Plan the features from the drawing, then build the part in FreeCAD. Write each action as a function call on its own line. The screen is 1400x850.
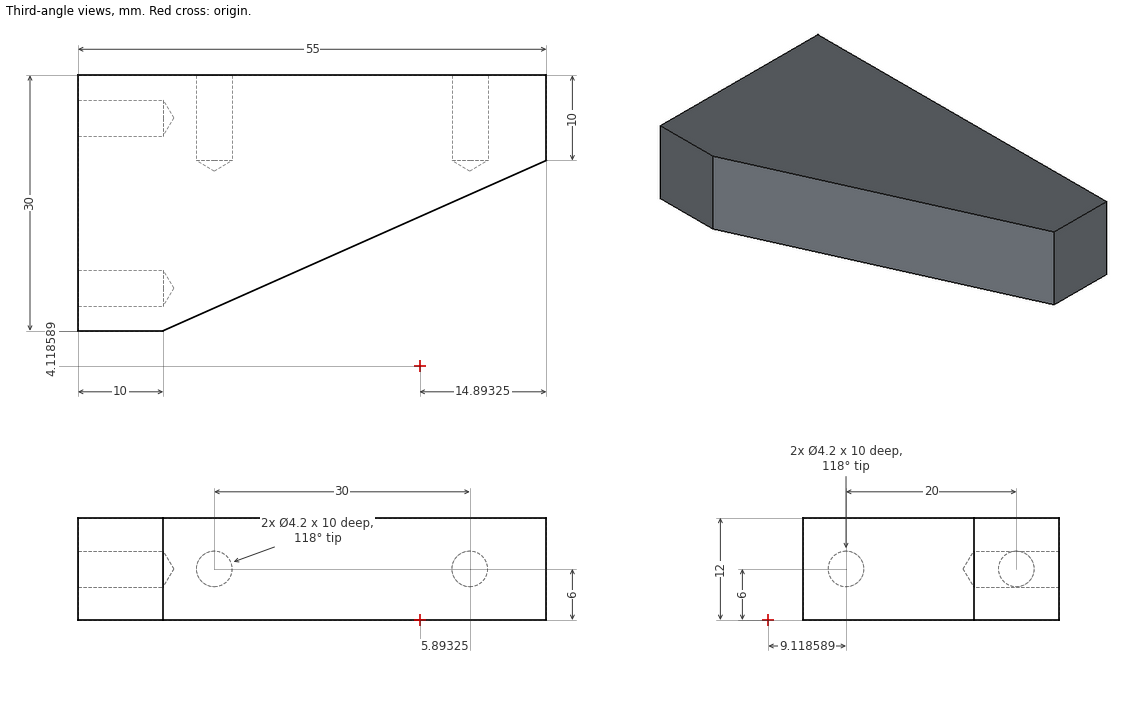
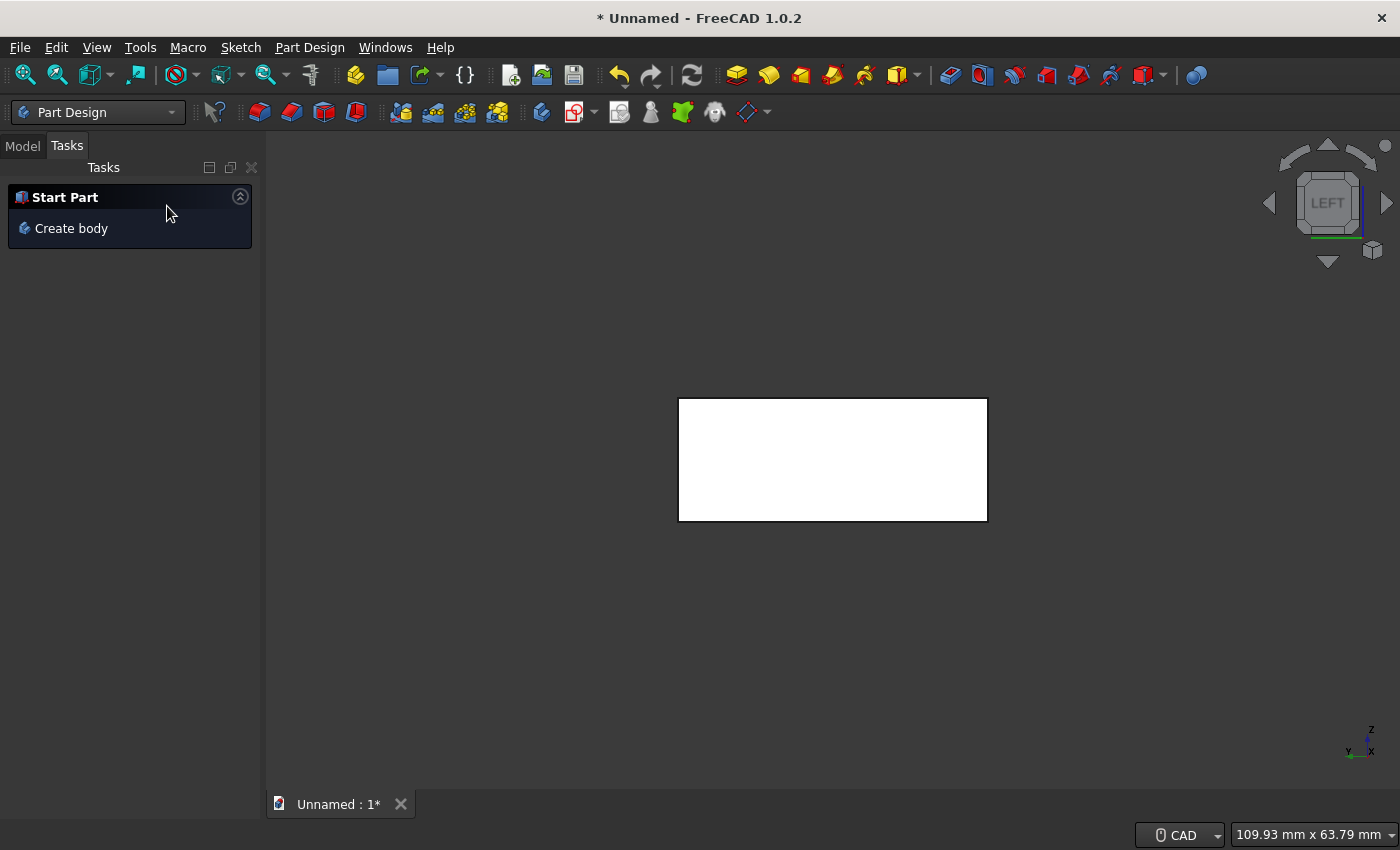
click(26, 76)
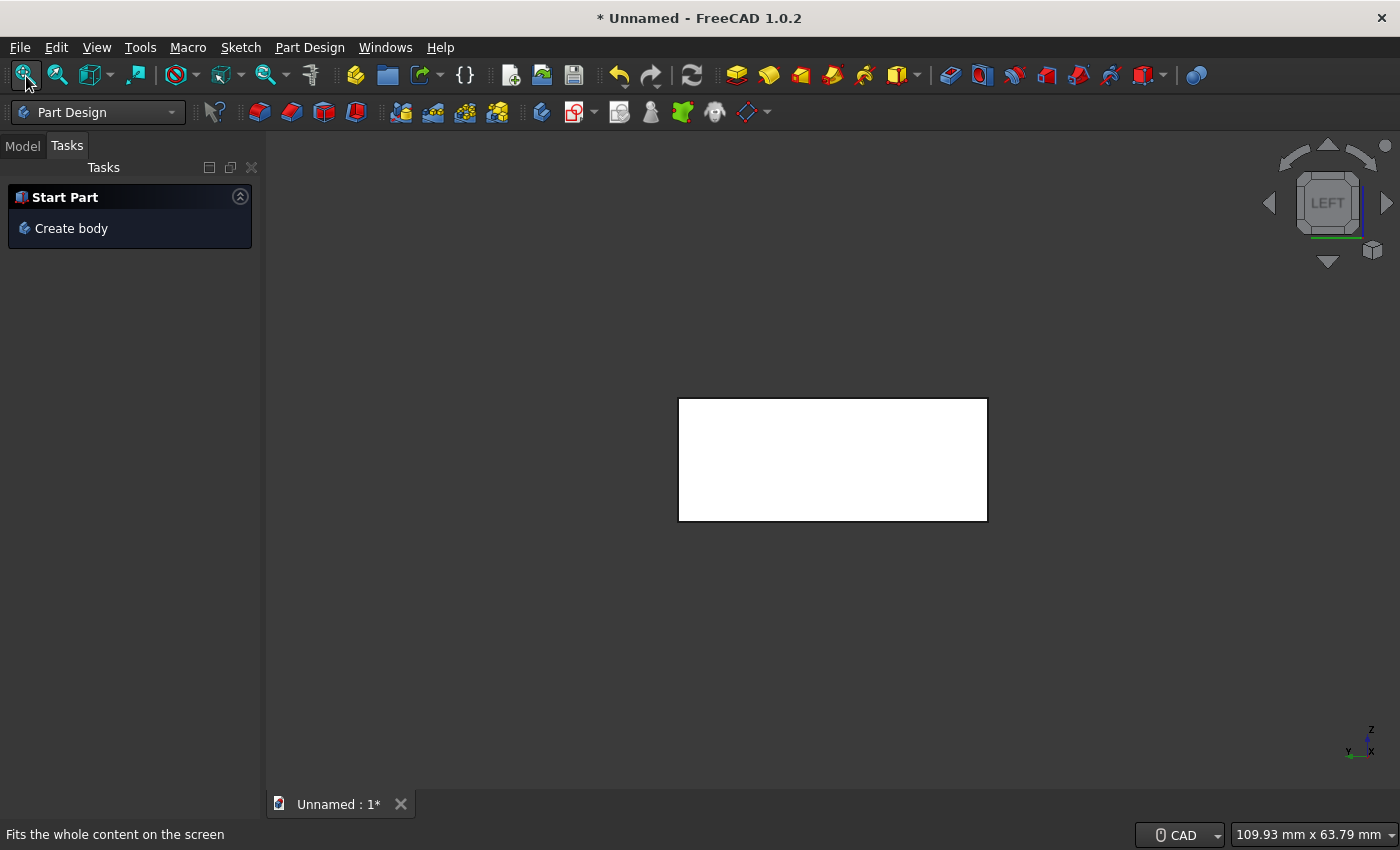
click(745, 459)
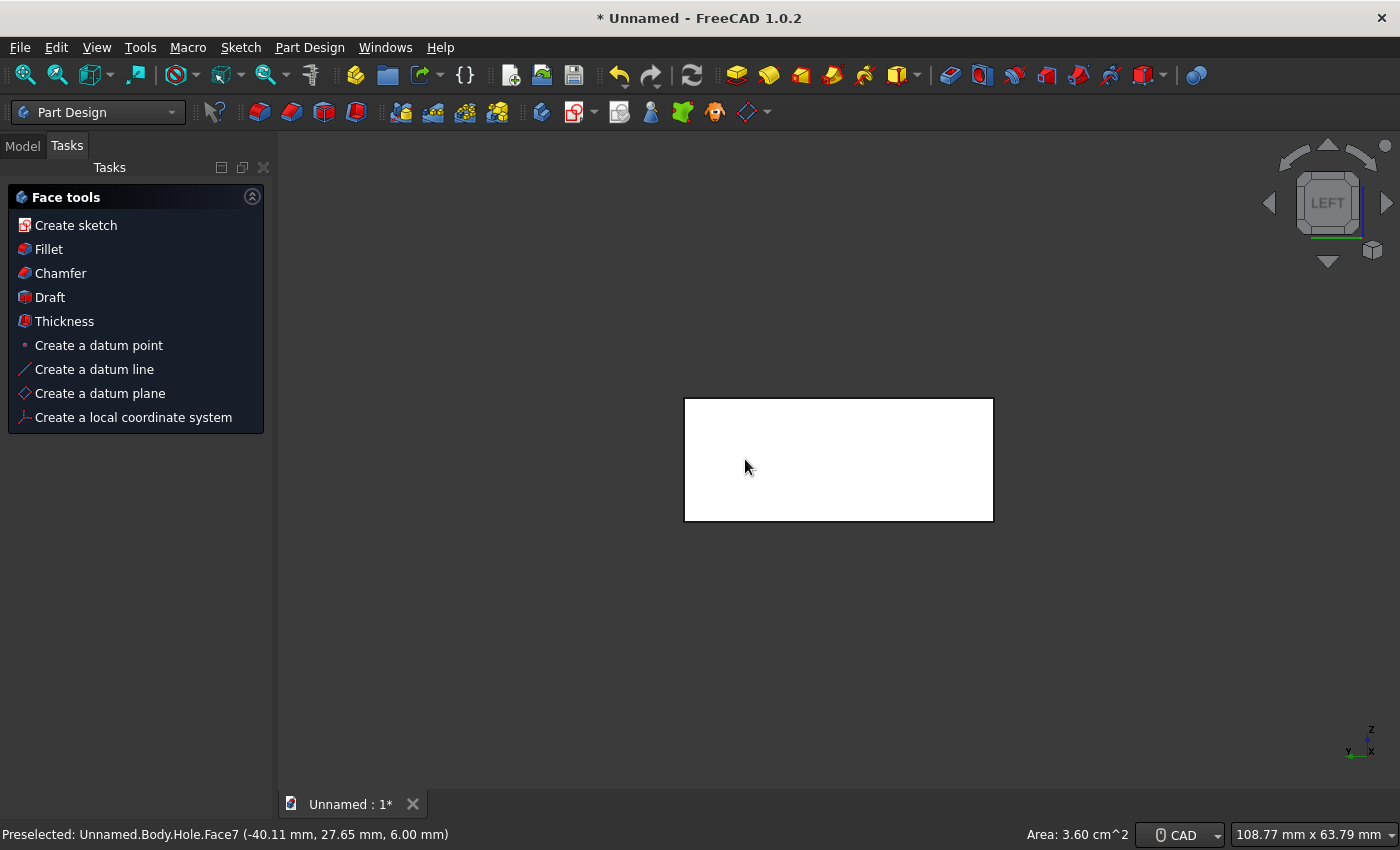
click(574, 112)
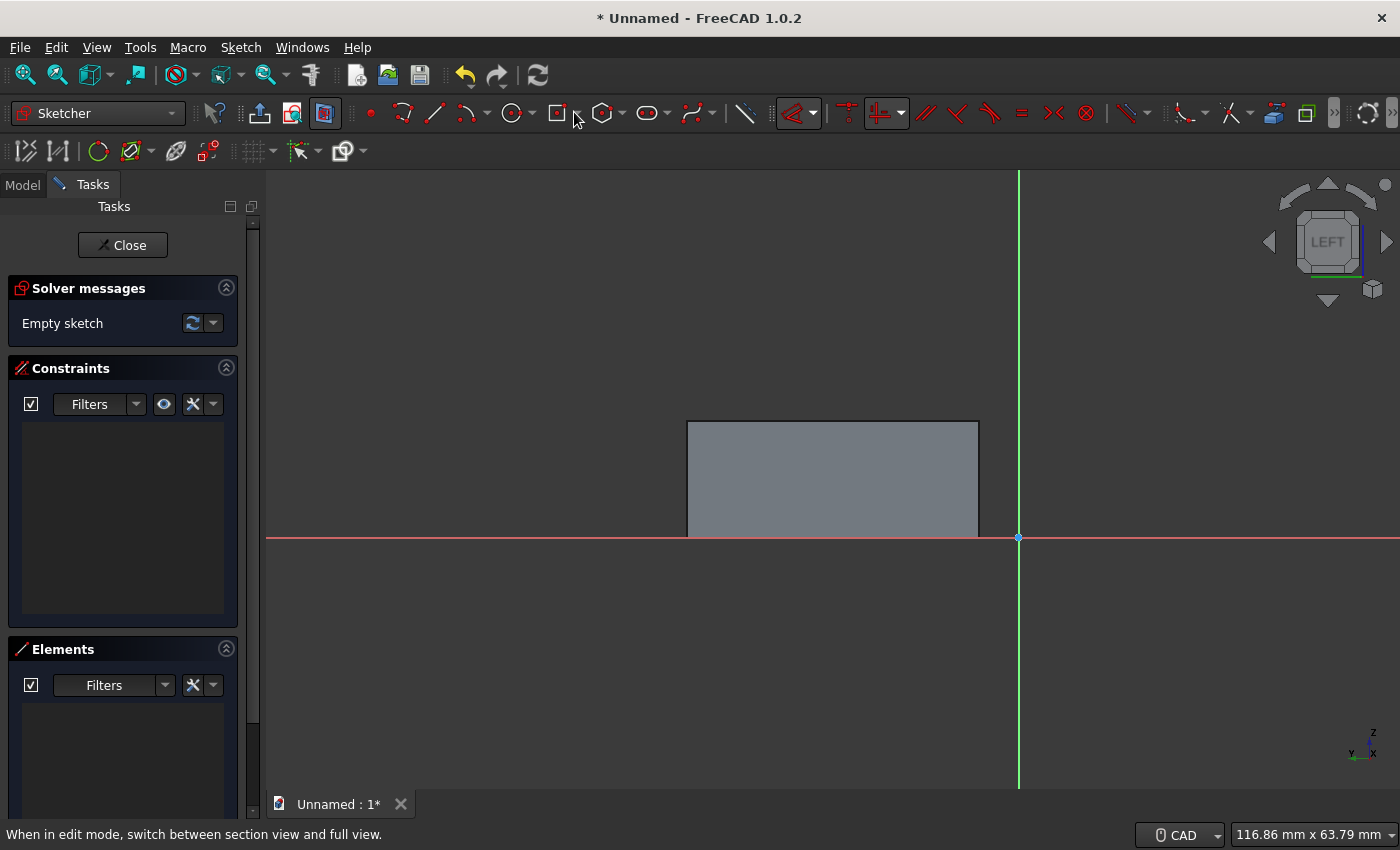
scroll(951, 514, up, 4)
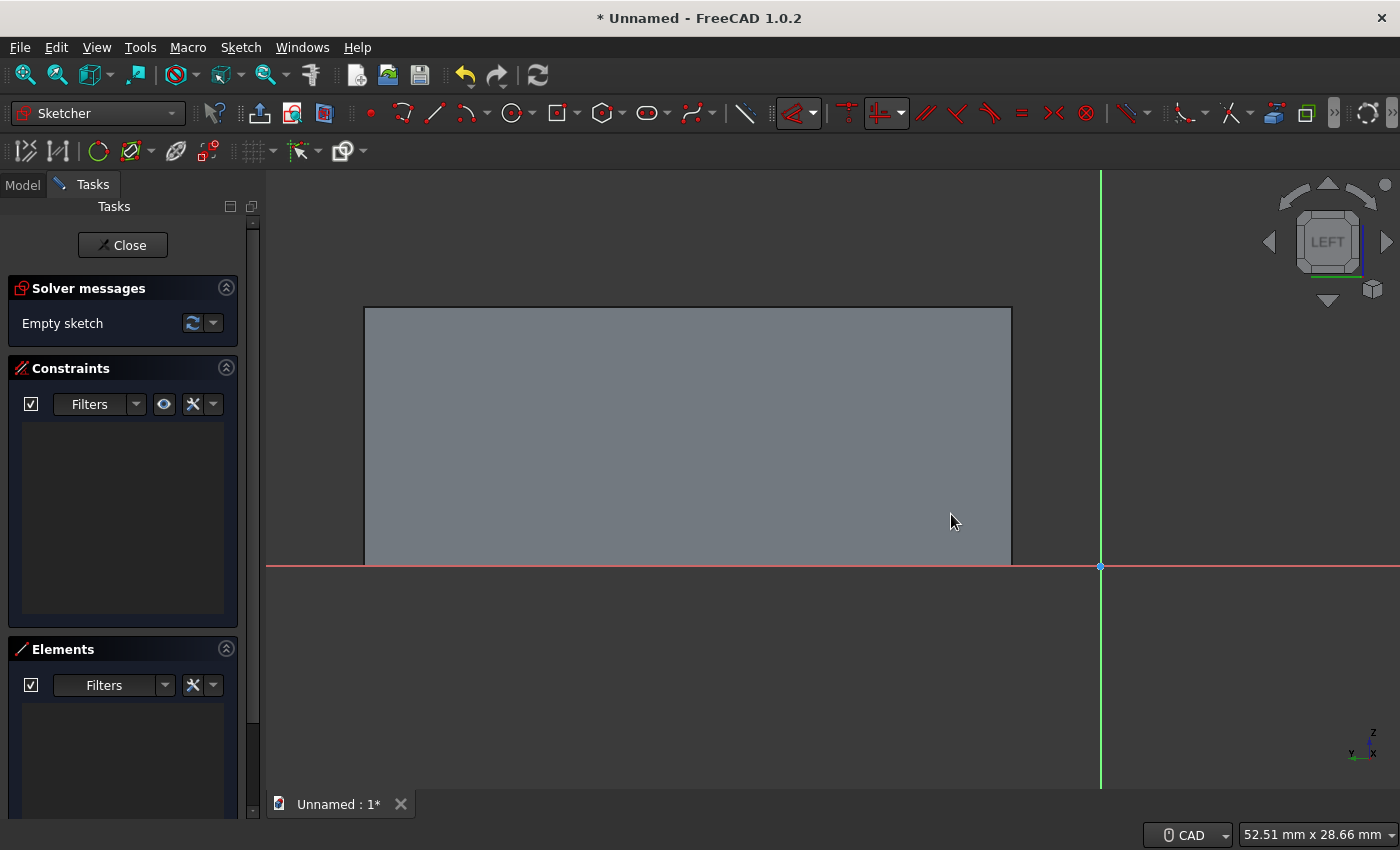
key(g)
key(c)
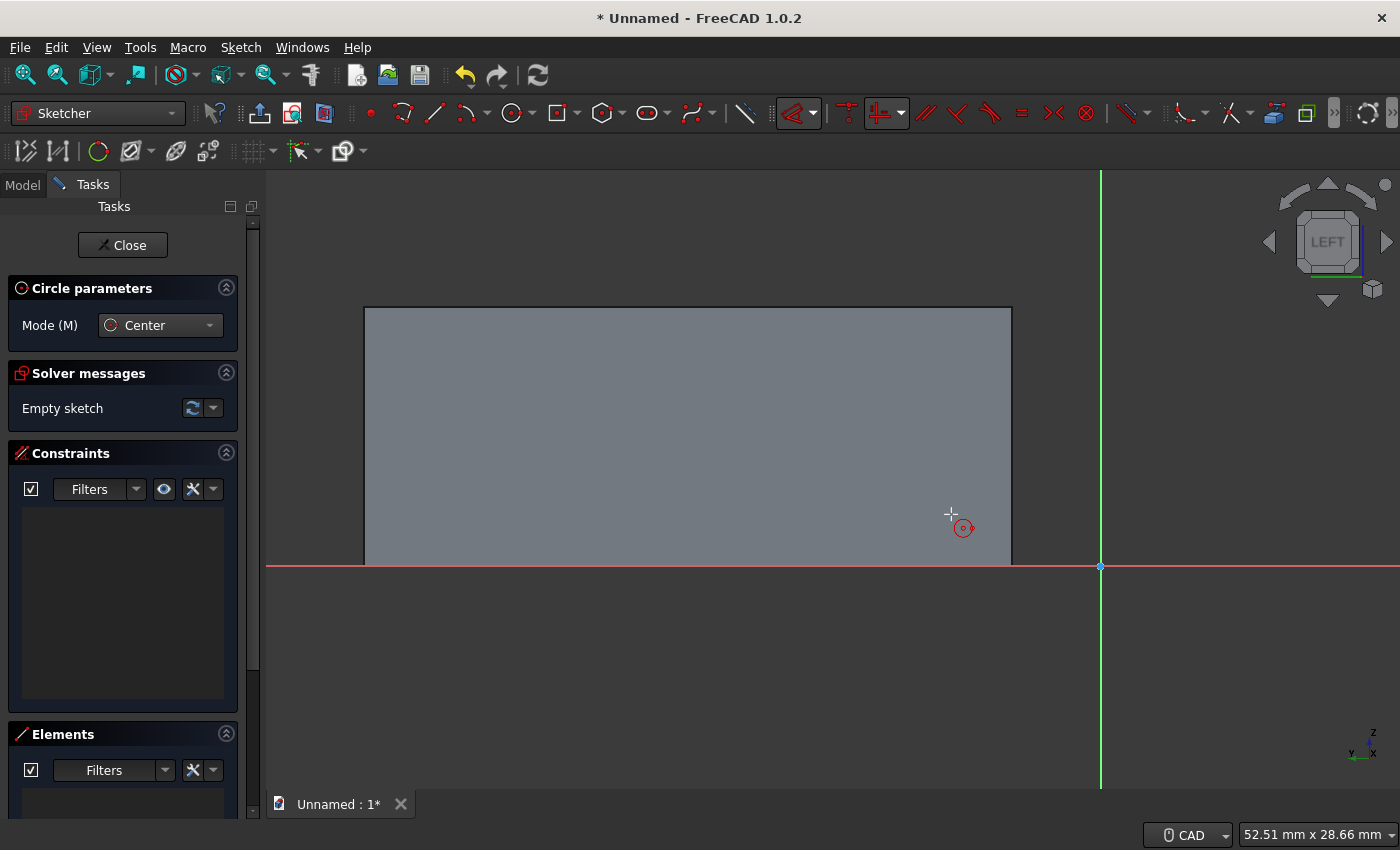
click(904, 437)
click(936, 404)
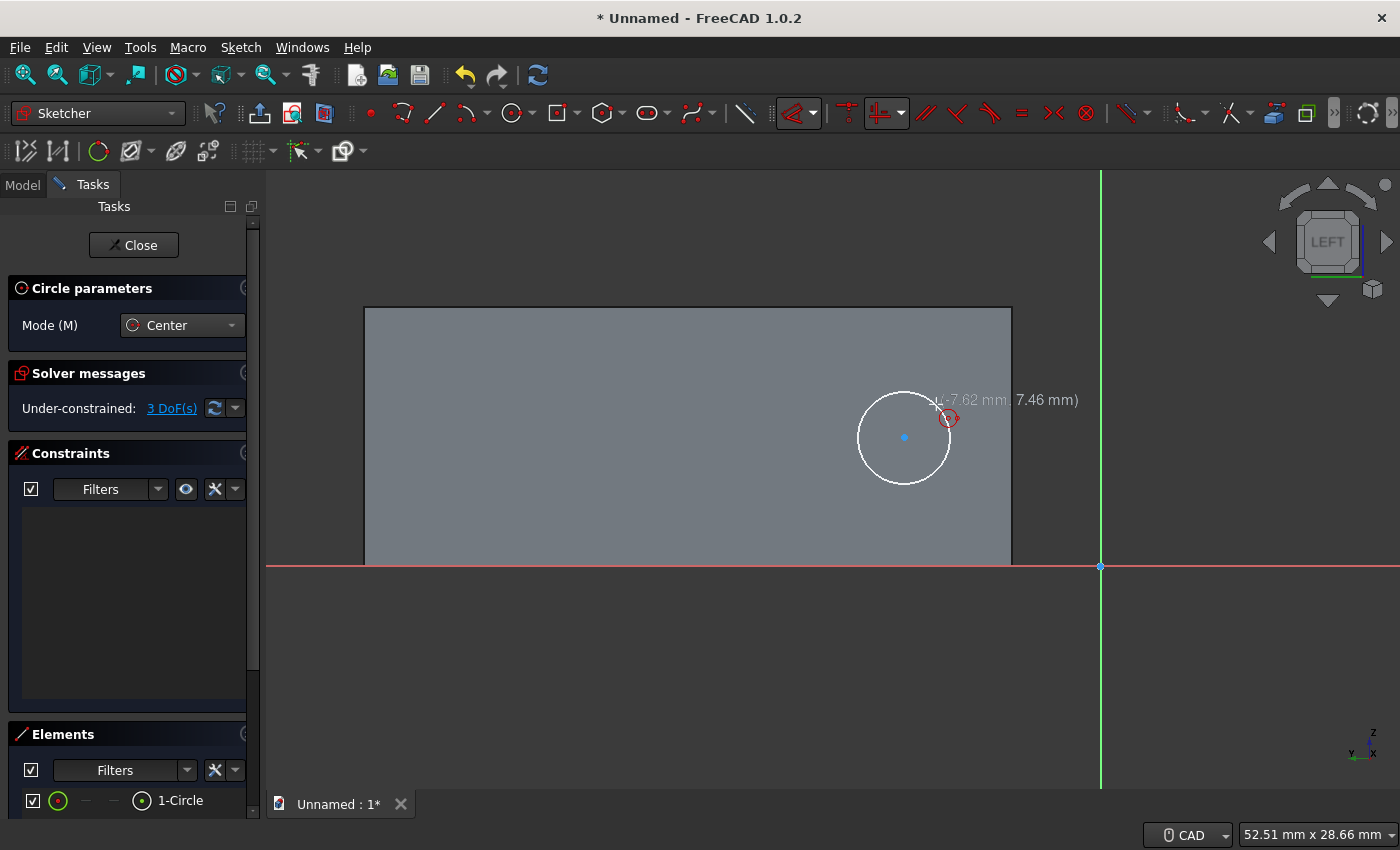
click(472, 437)
click(504, 404)
key(Escape)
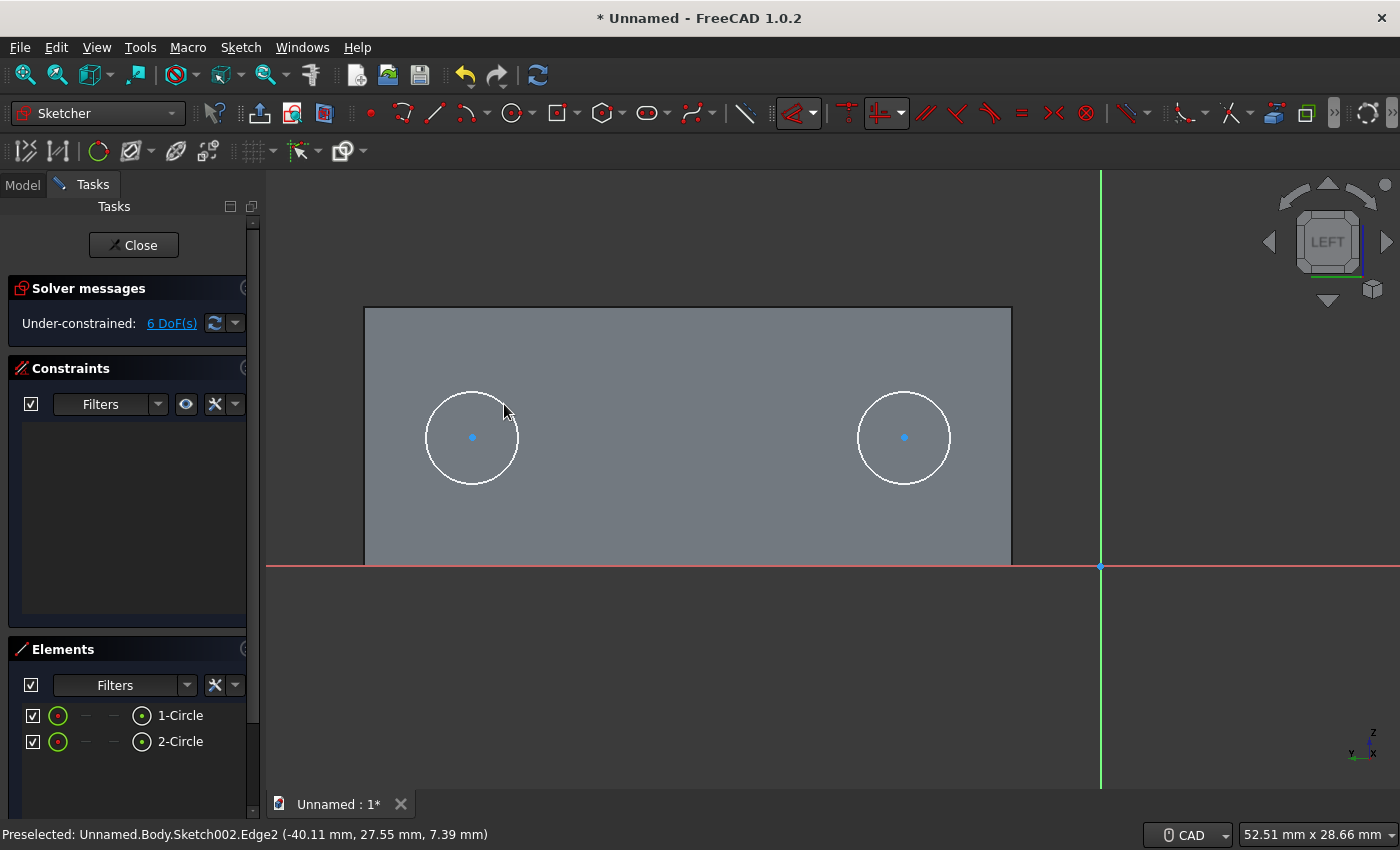
click(936, 405)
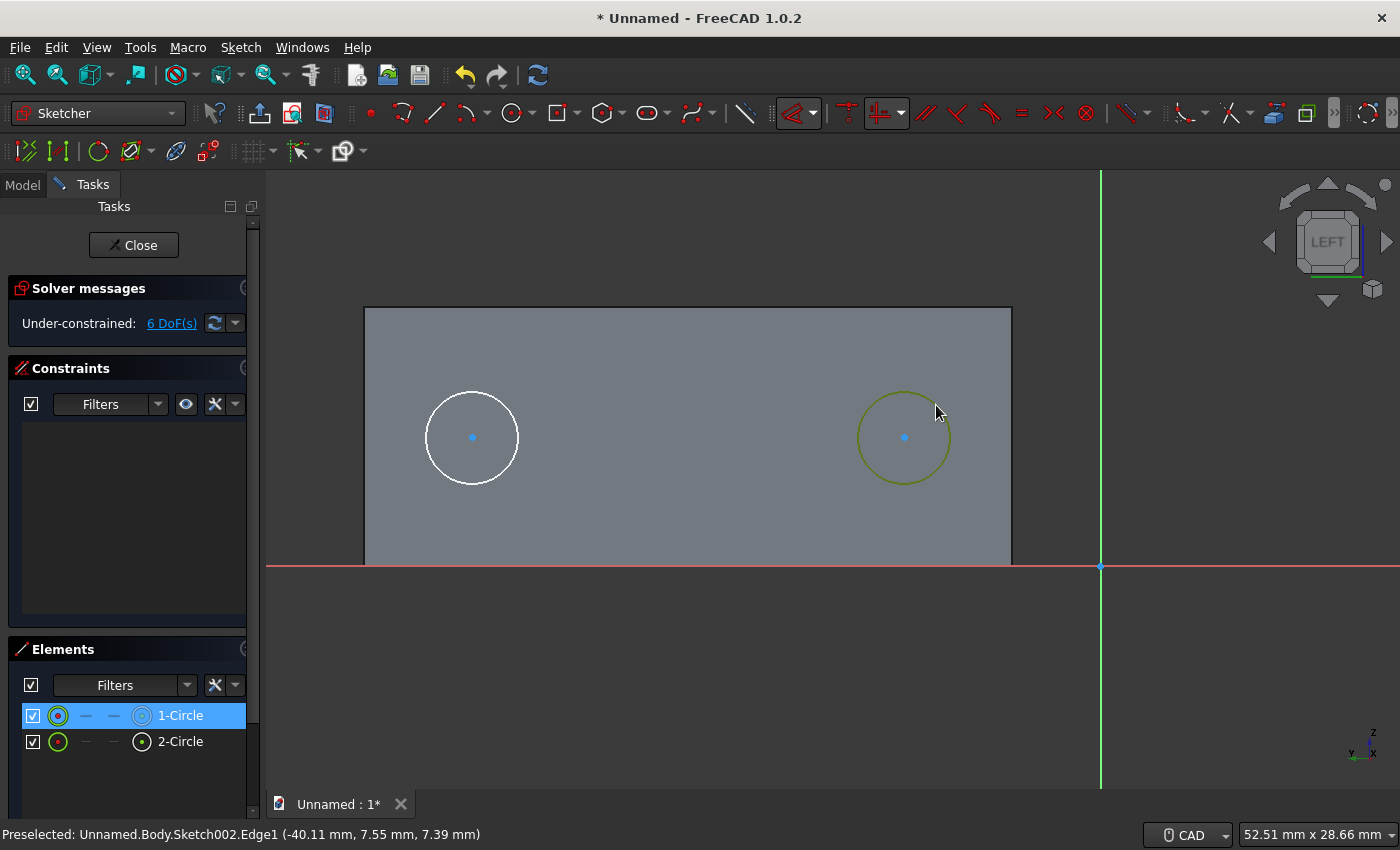
click(504, 405)